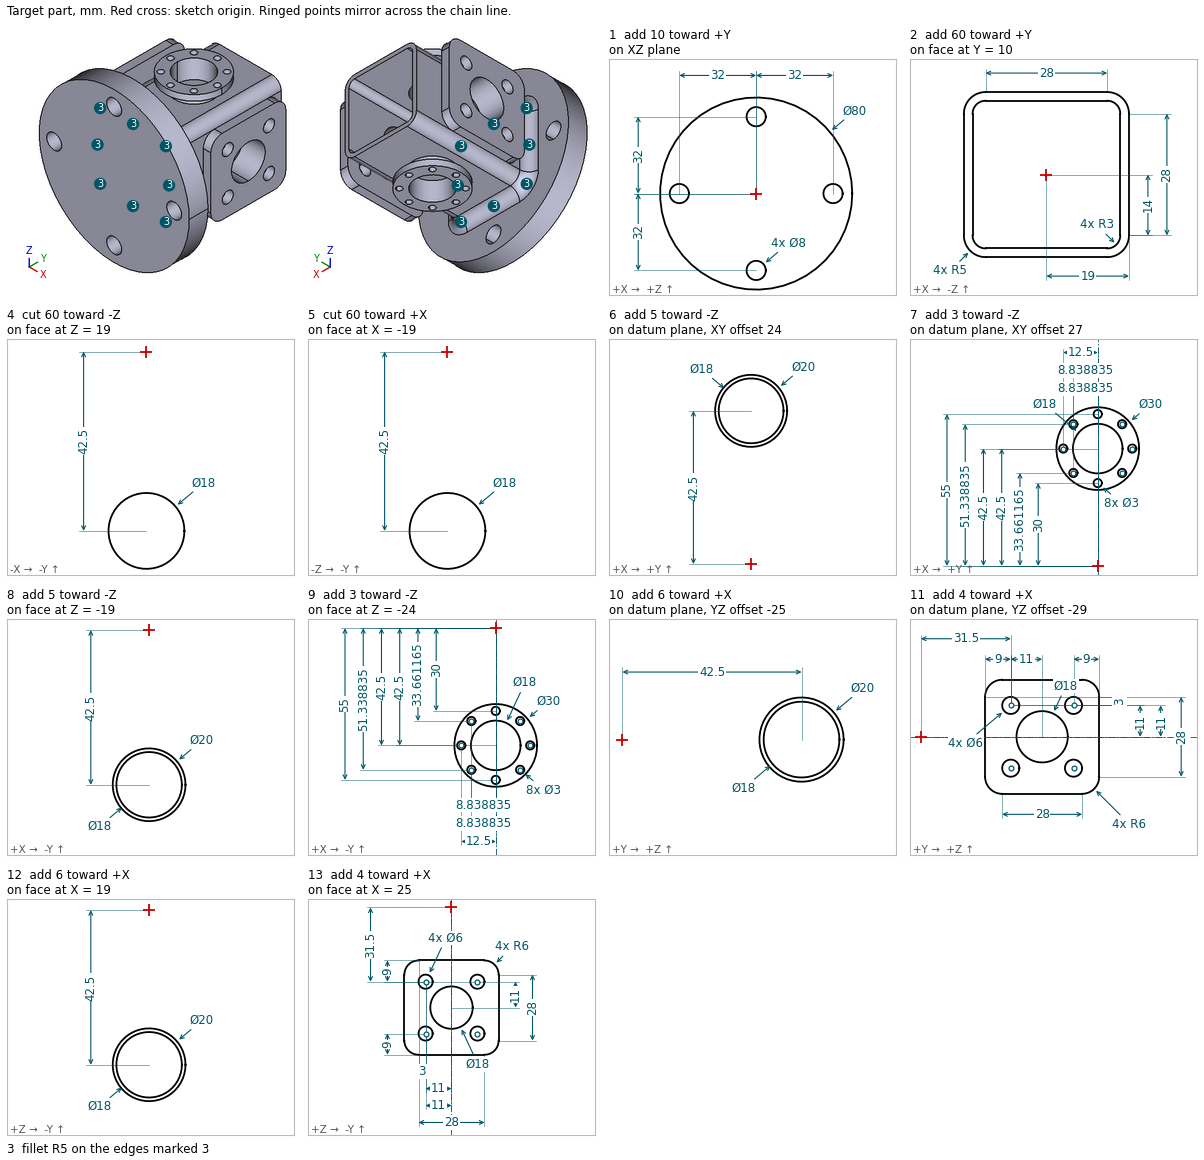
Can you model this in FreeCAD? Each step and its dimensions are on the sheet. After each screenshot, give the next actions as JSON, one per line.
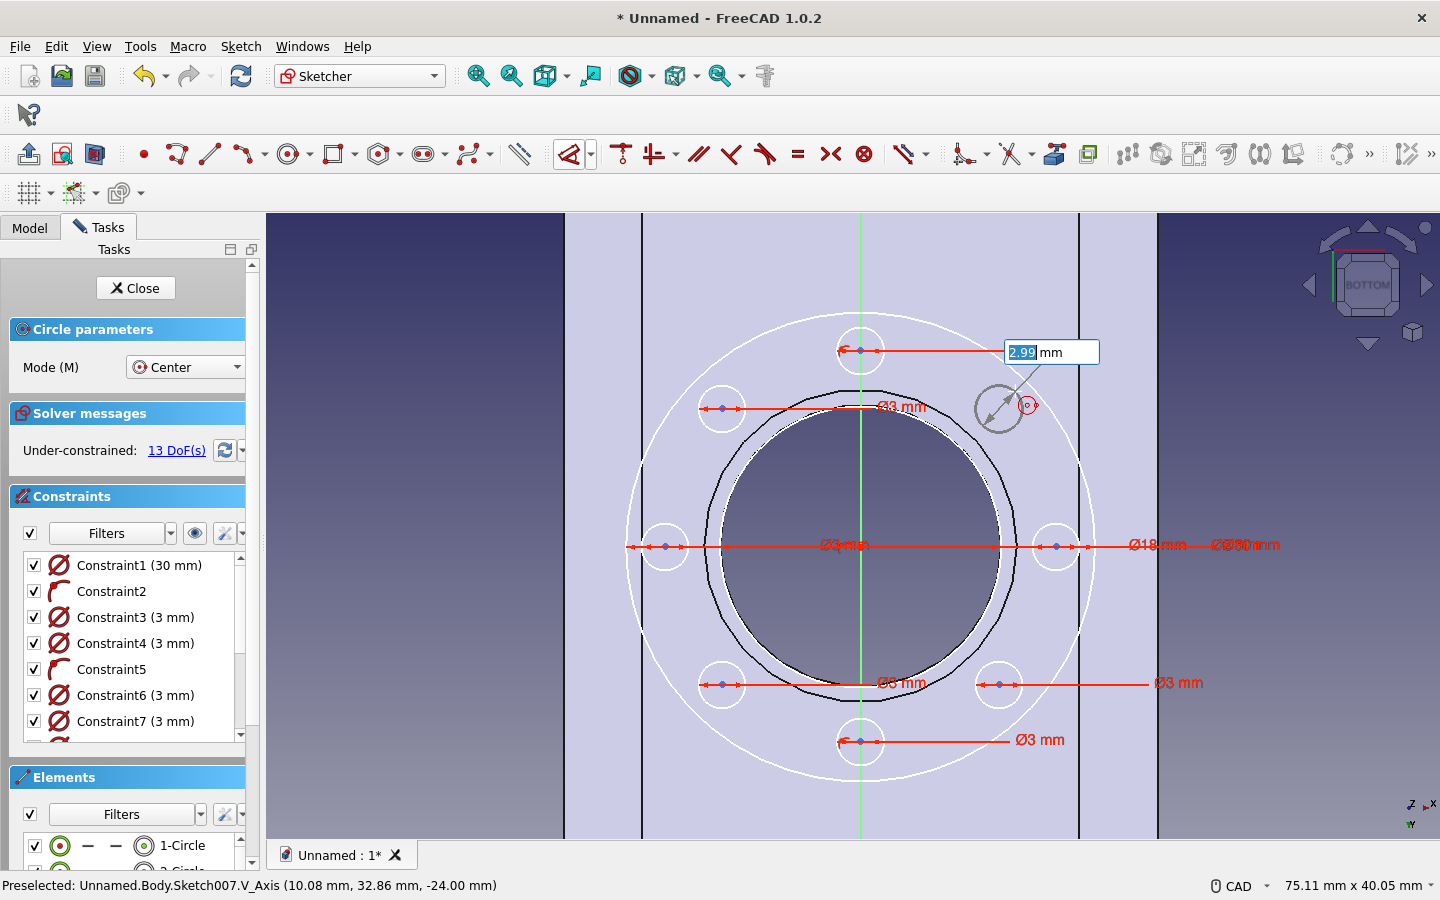
{"action": "type", "text": "3"}
{"action": "key", "text": "Return"}
{"action": "key", "text": "Escape"}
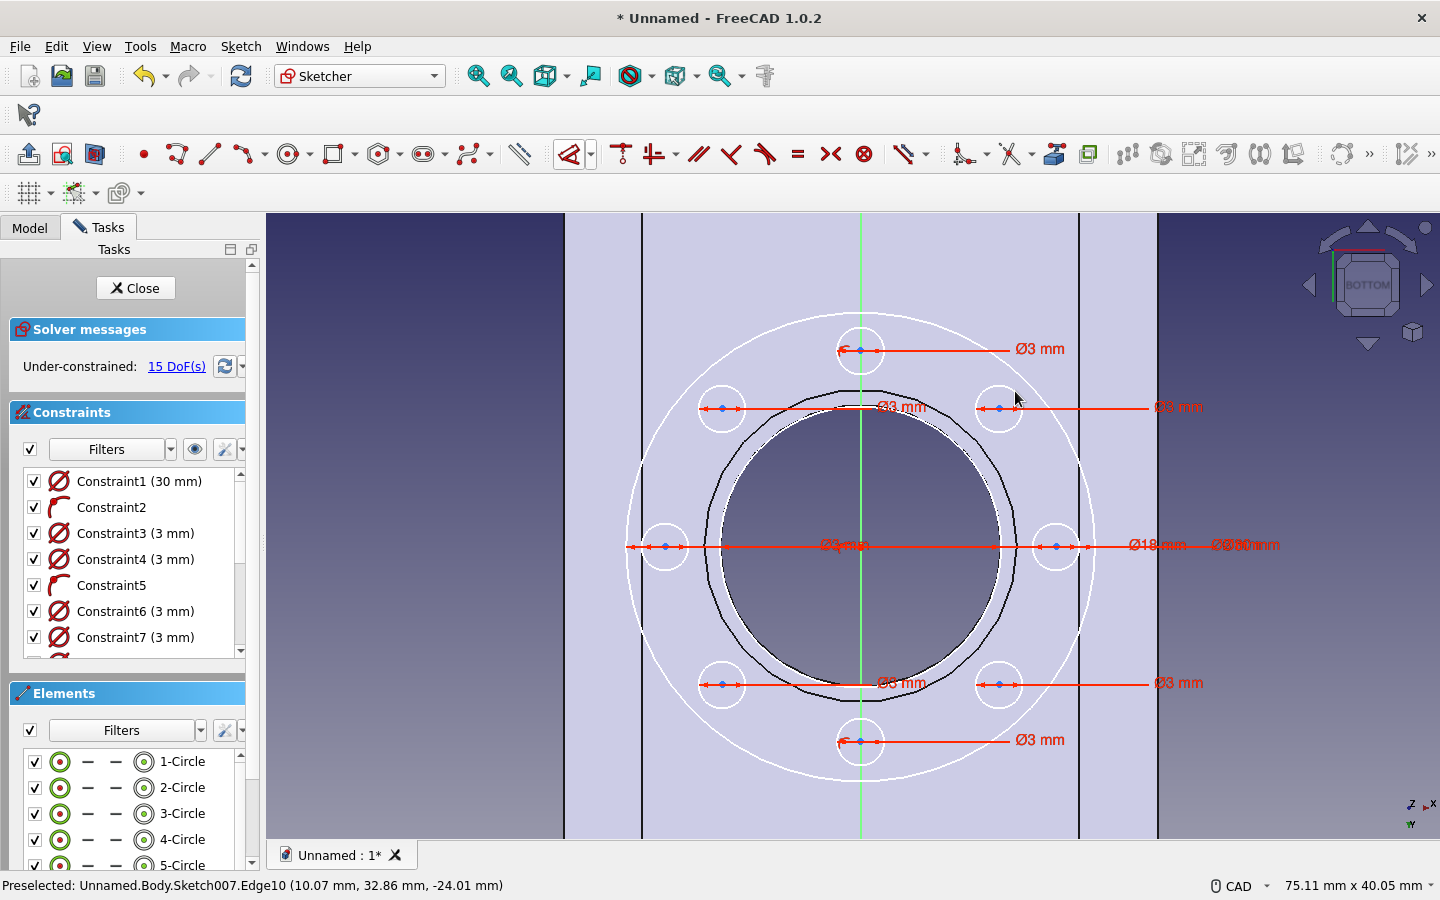
{"action": "left_click", "coordinate": [722, 685]}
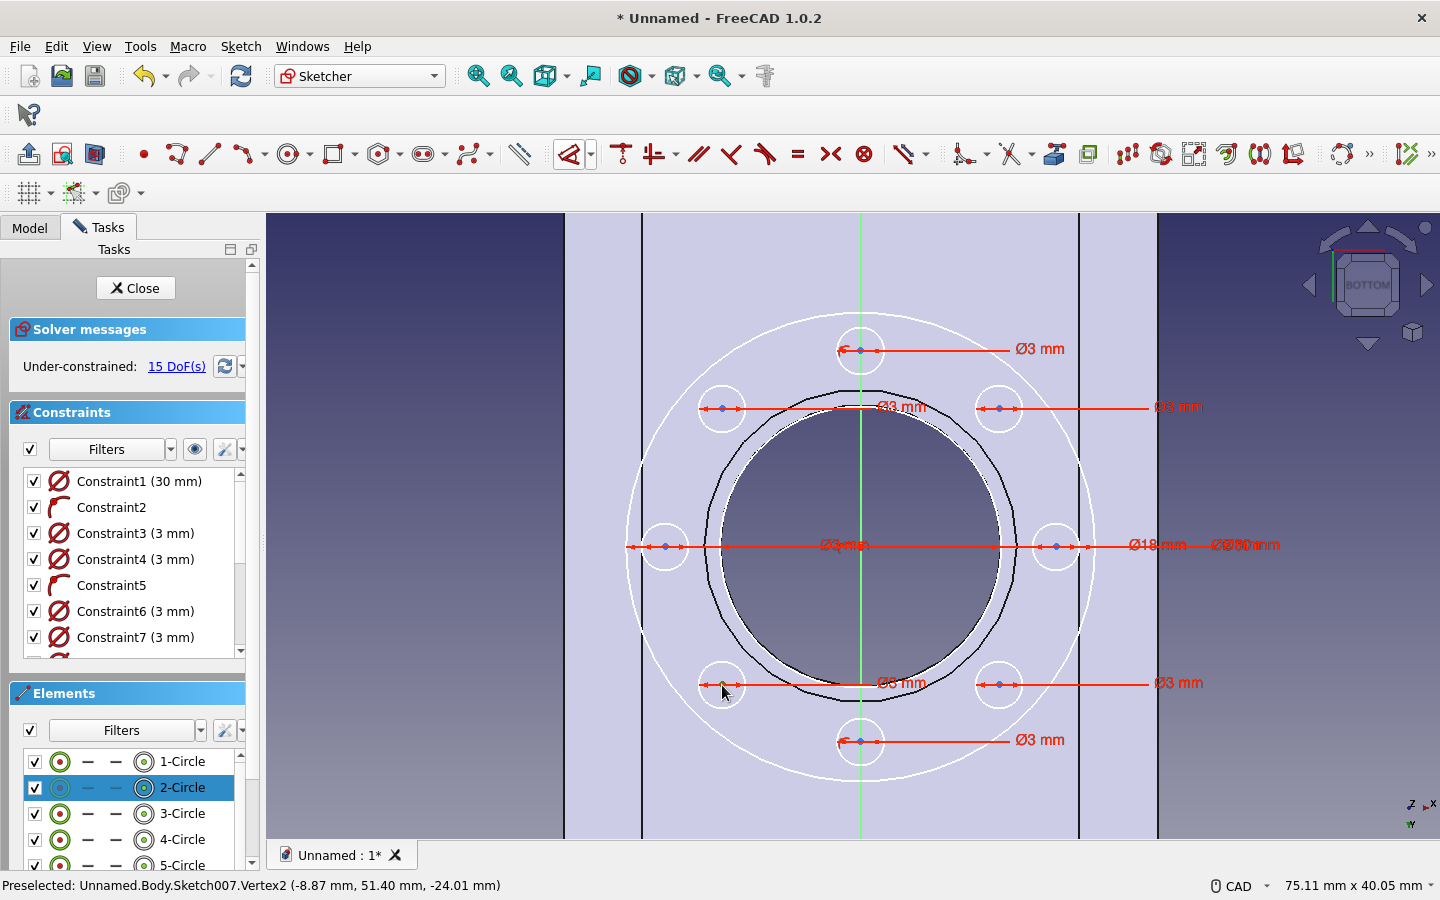
{"action": "left_click", "coordinate": [999, 685]}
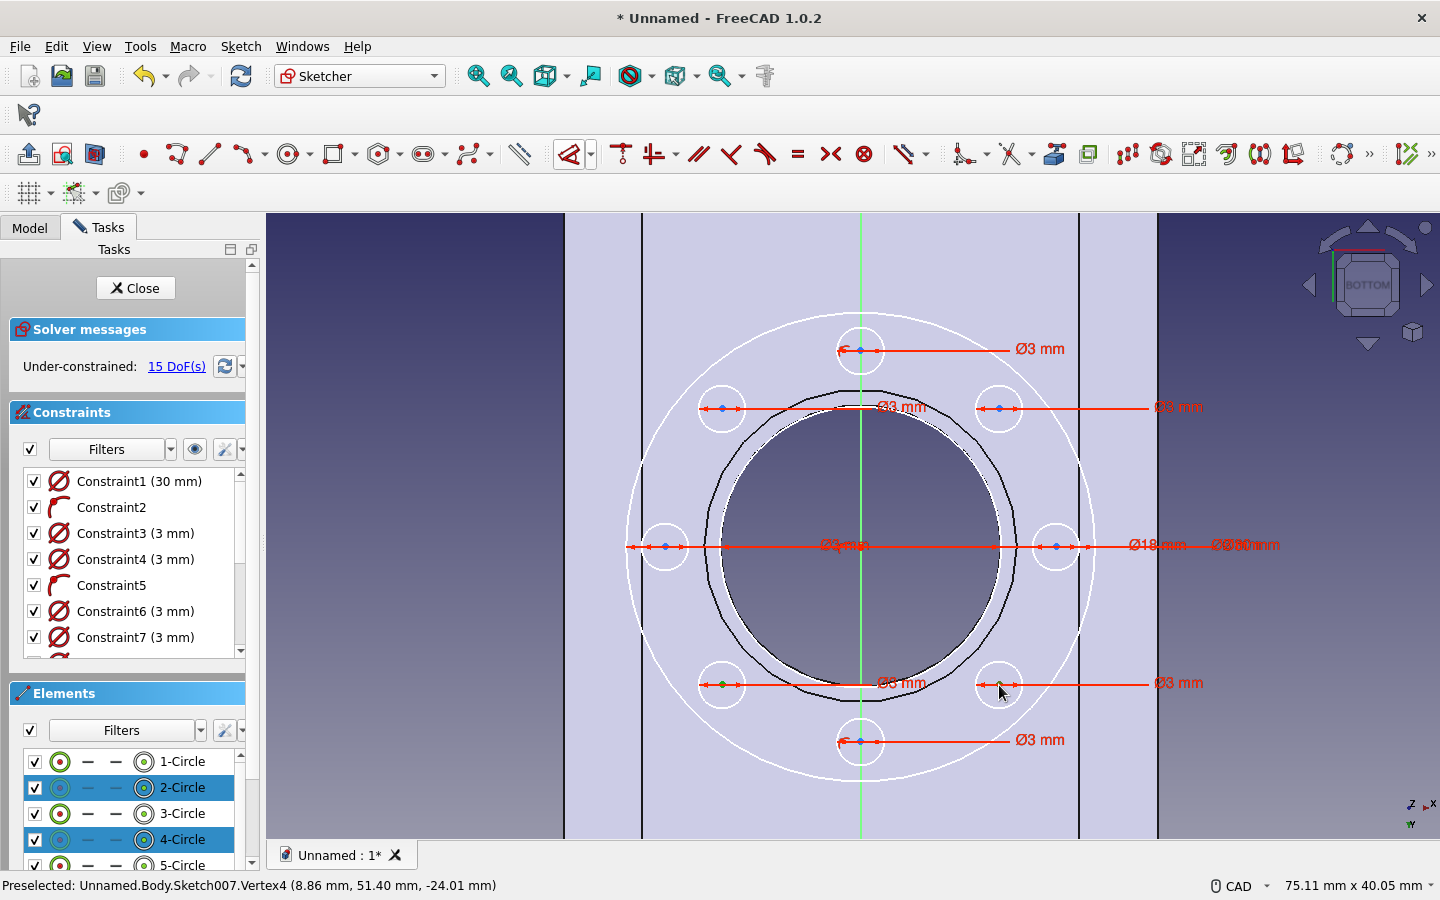
{"action": "left_click", "coordinate": [861, 648]}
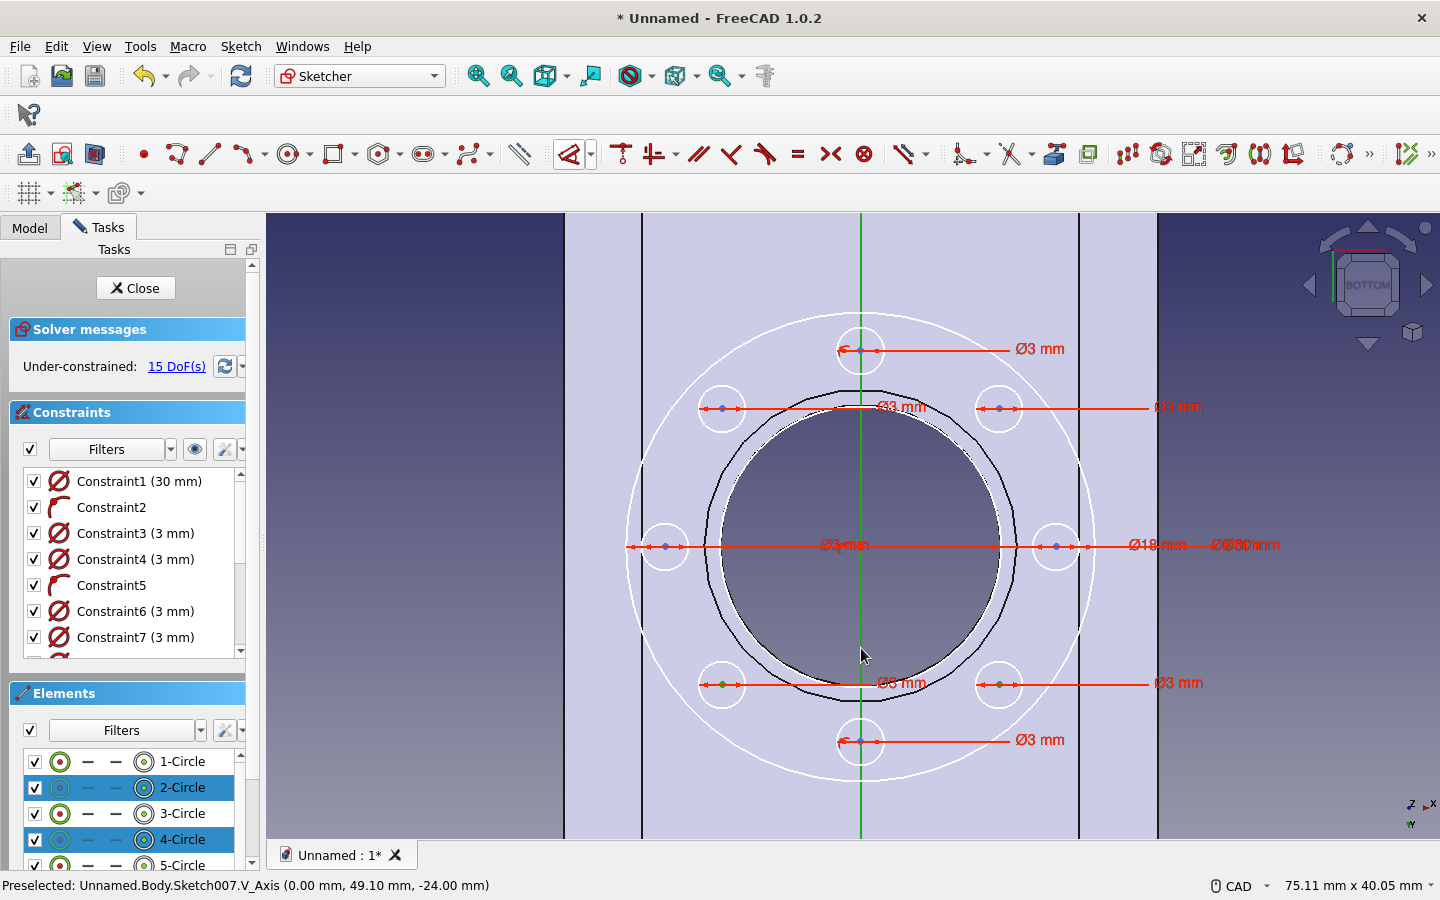
{"action": "key", "text": "s"}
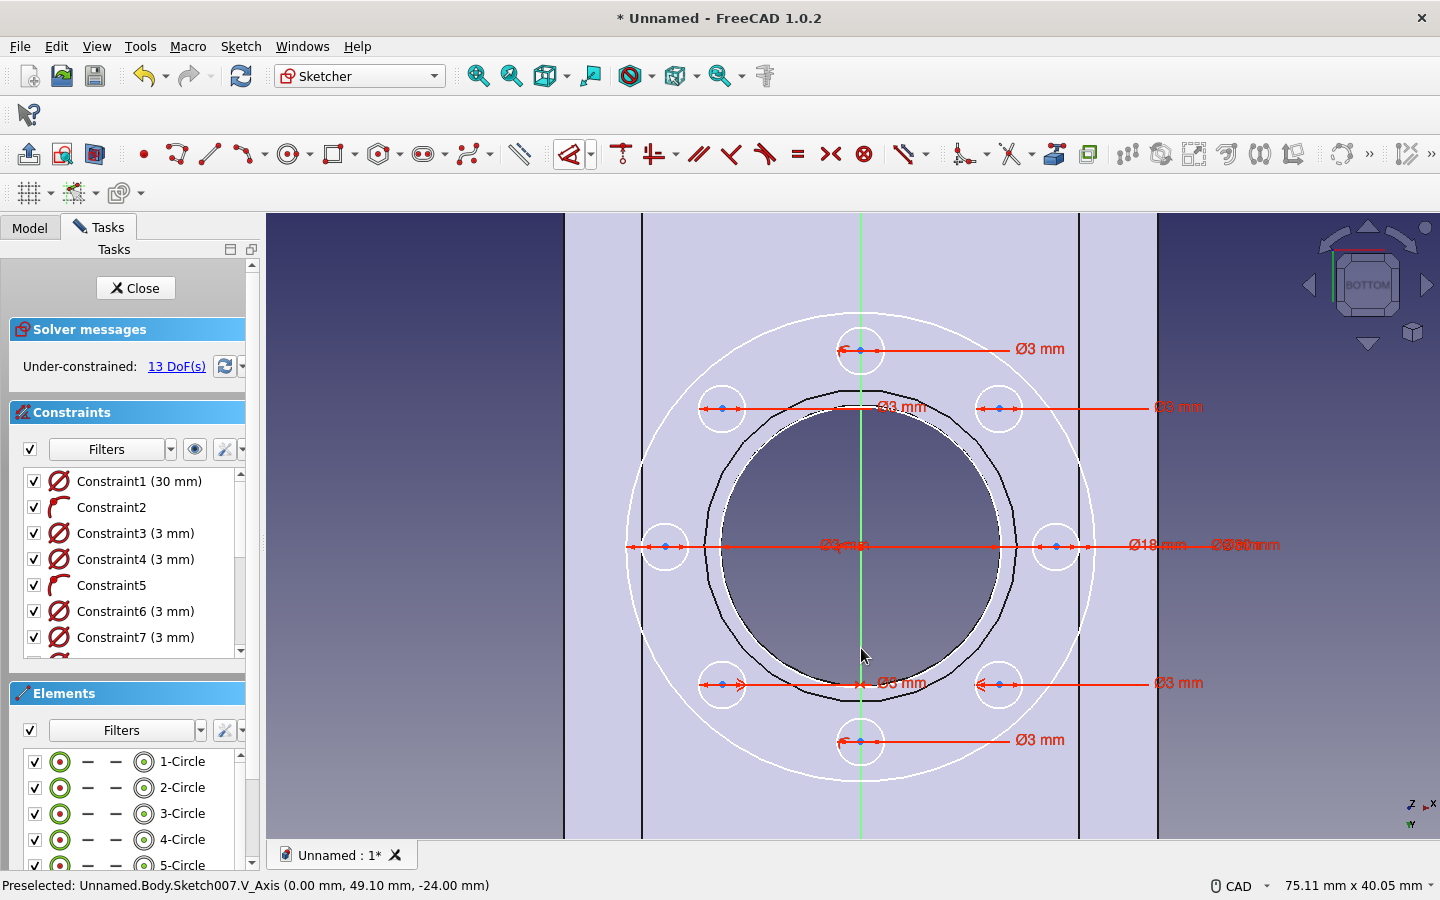
{"action": "left_click", "coordinate": [665, 547]}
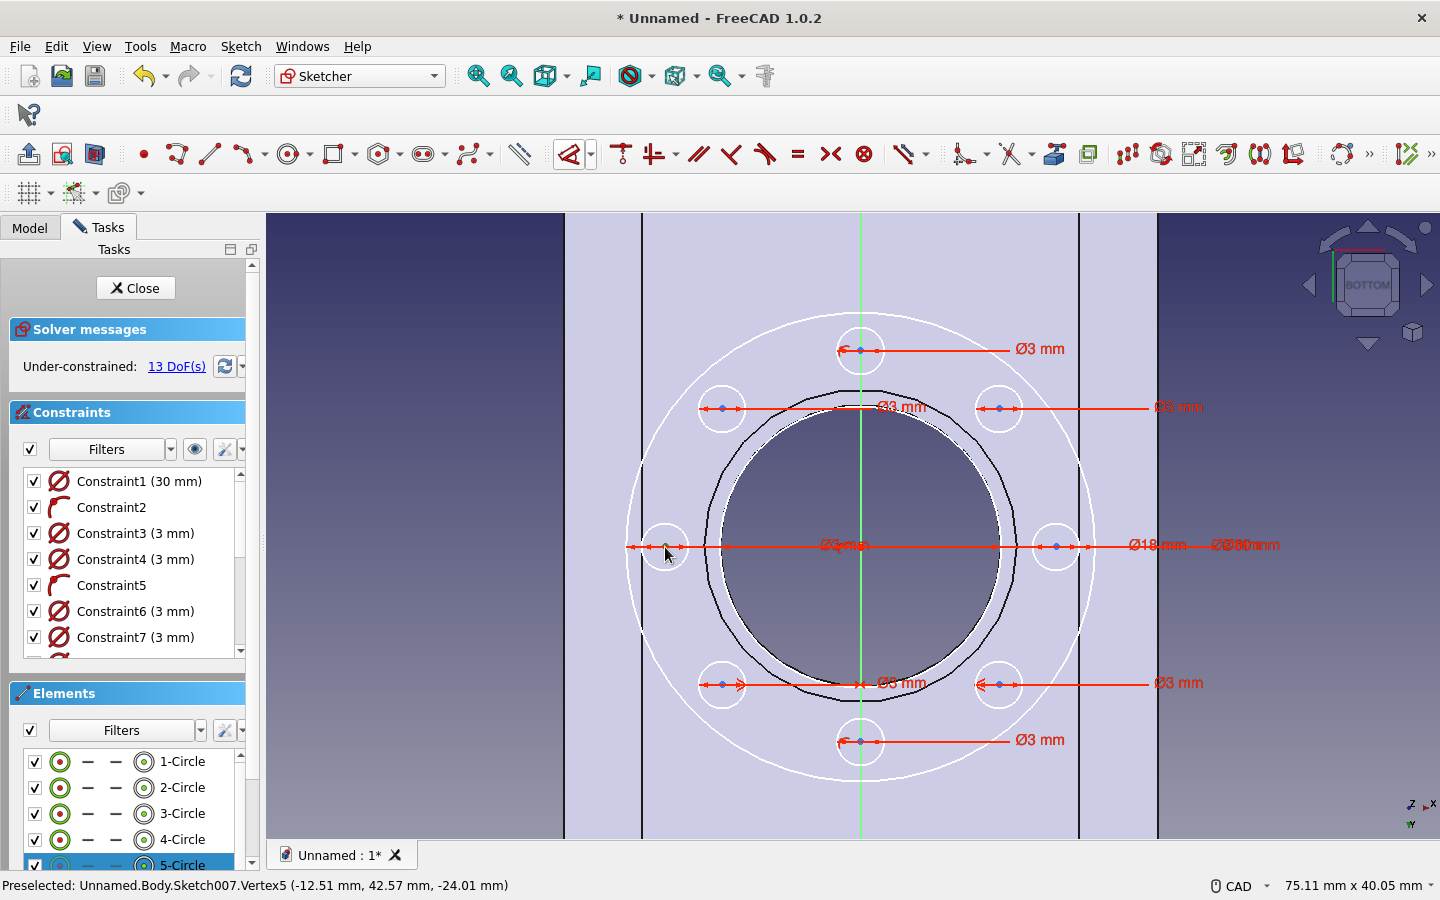
{"action": "left_click", "coordinate": [1056, 547]}